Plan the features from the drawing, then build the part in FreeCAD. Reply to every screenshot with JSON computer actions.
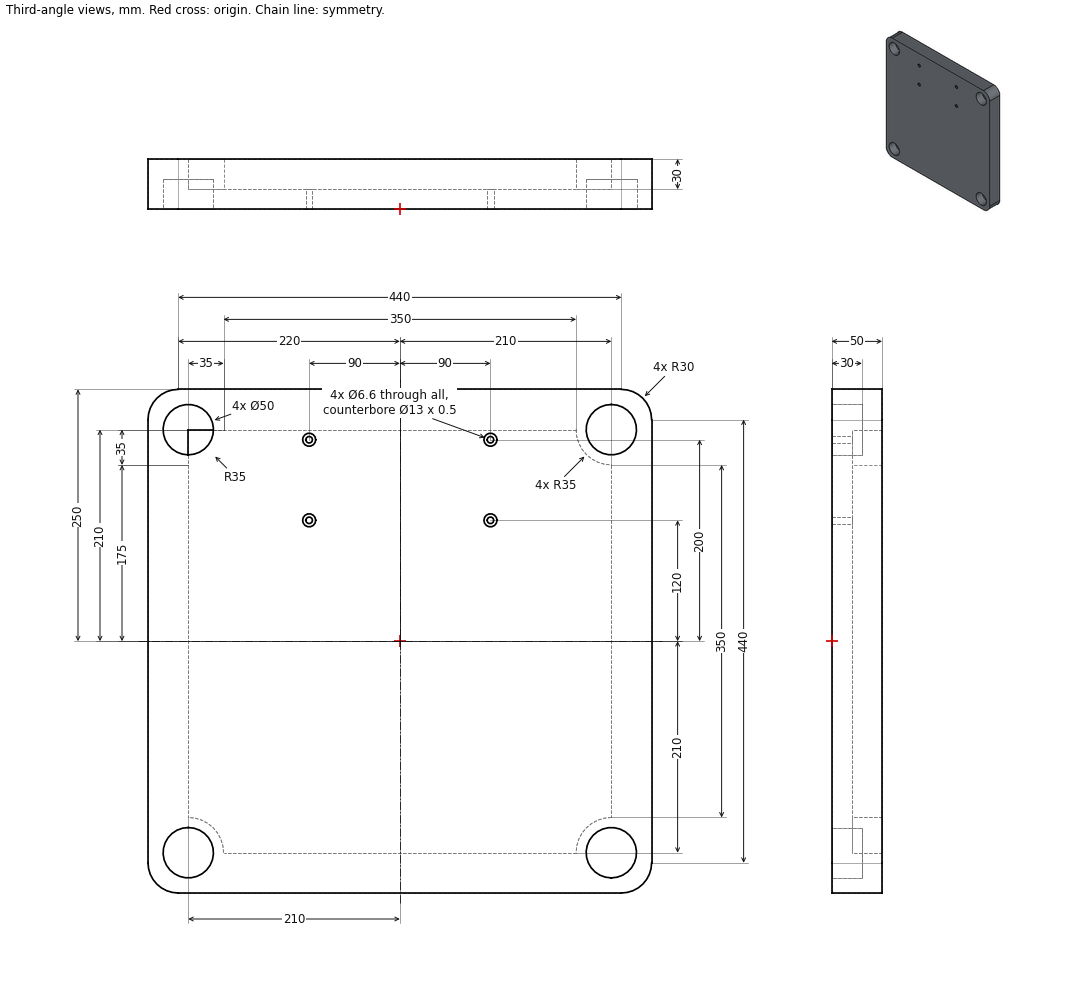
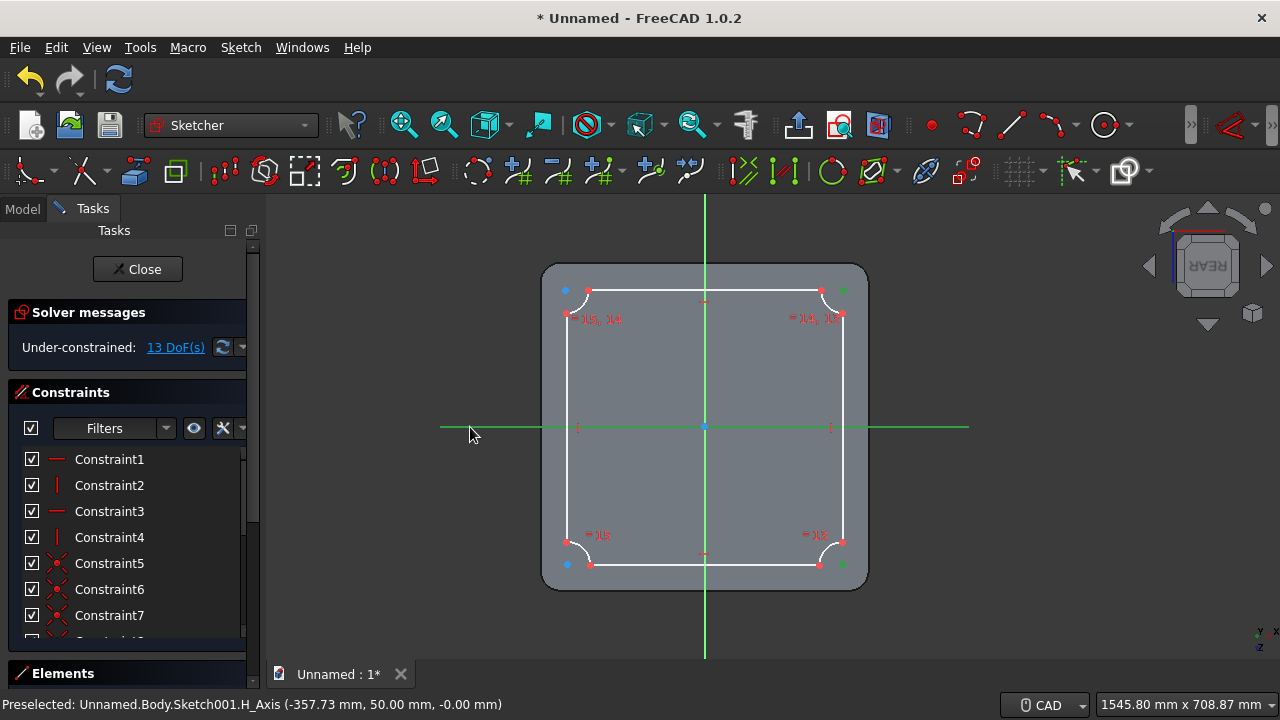
{"action": "key", "text": "s"}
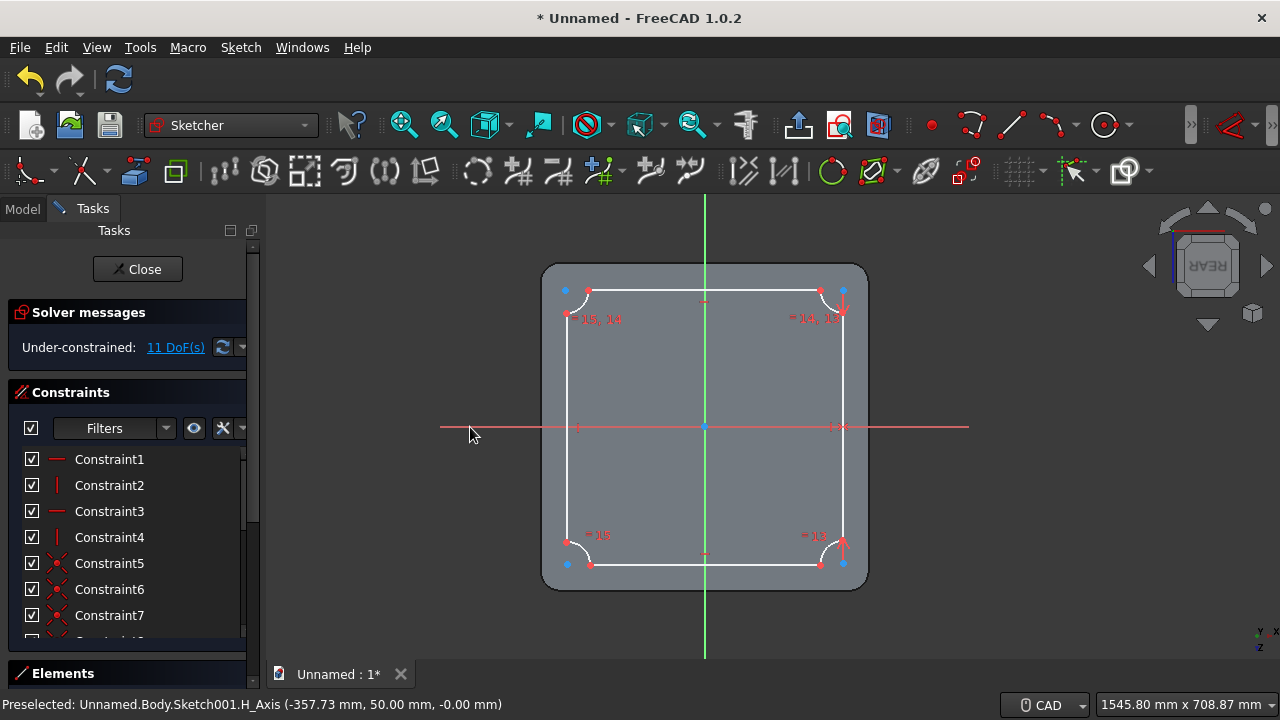
{"action": "left_click", "coordinate": [843, 290]}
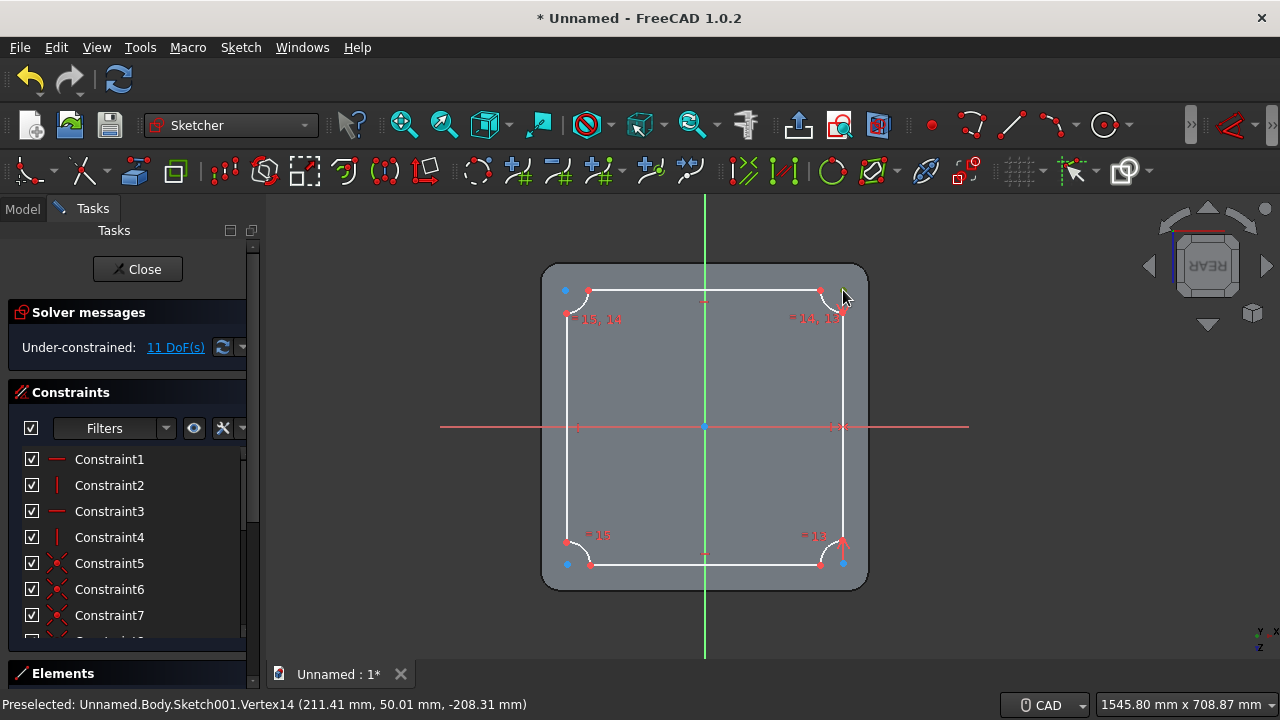
{"action": "left_click", "coordinate": [566, 291]}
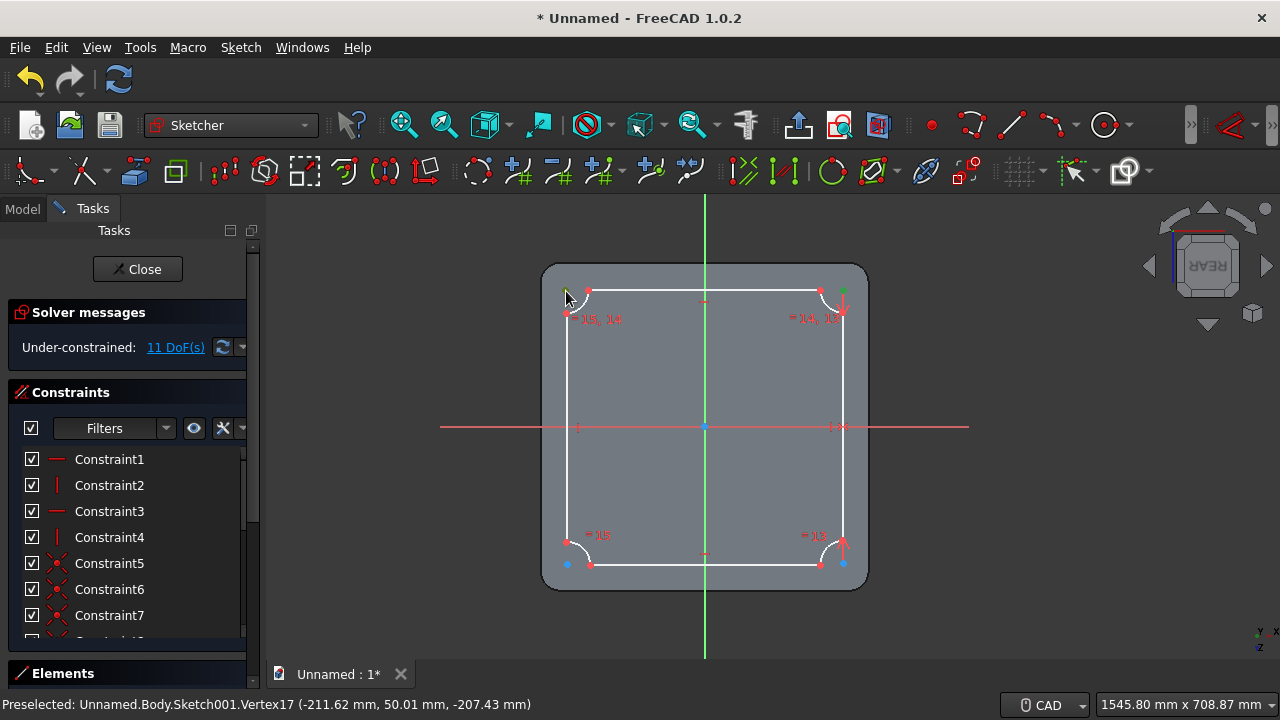
{"action": "left_click", "coordinate": [705, 602]}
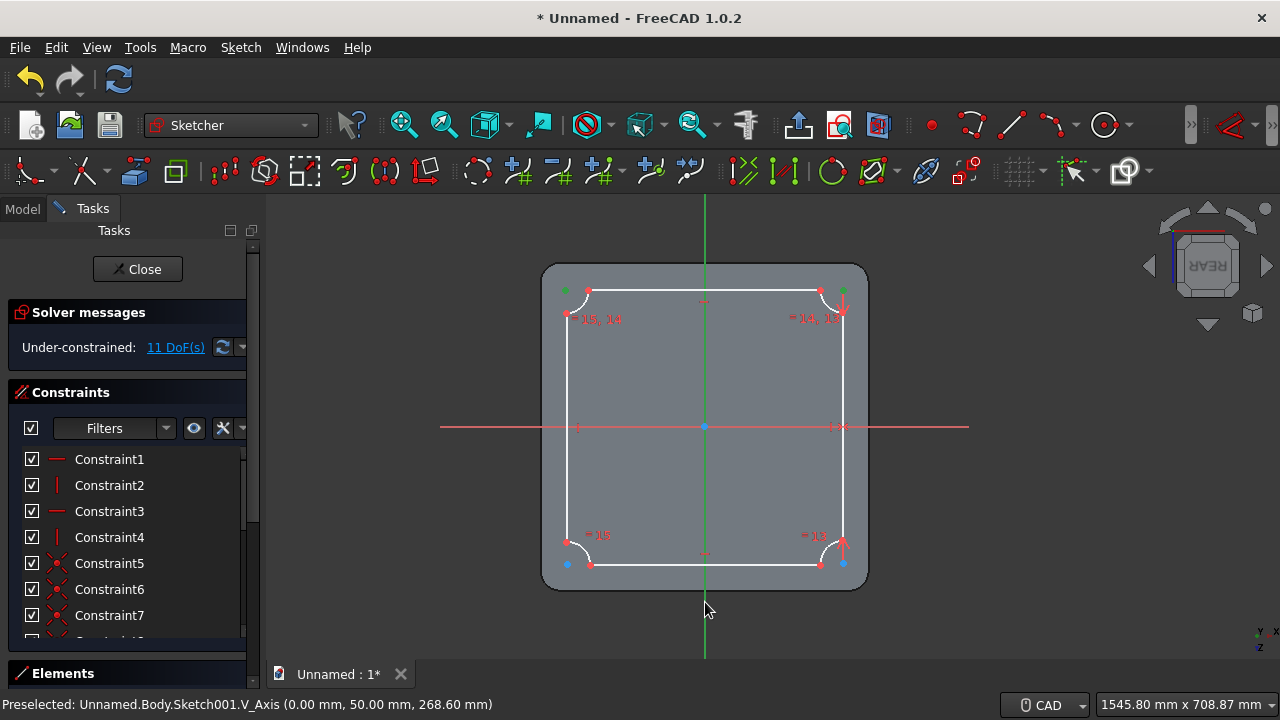
{"action": "key", "text": "s"}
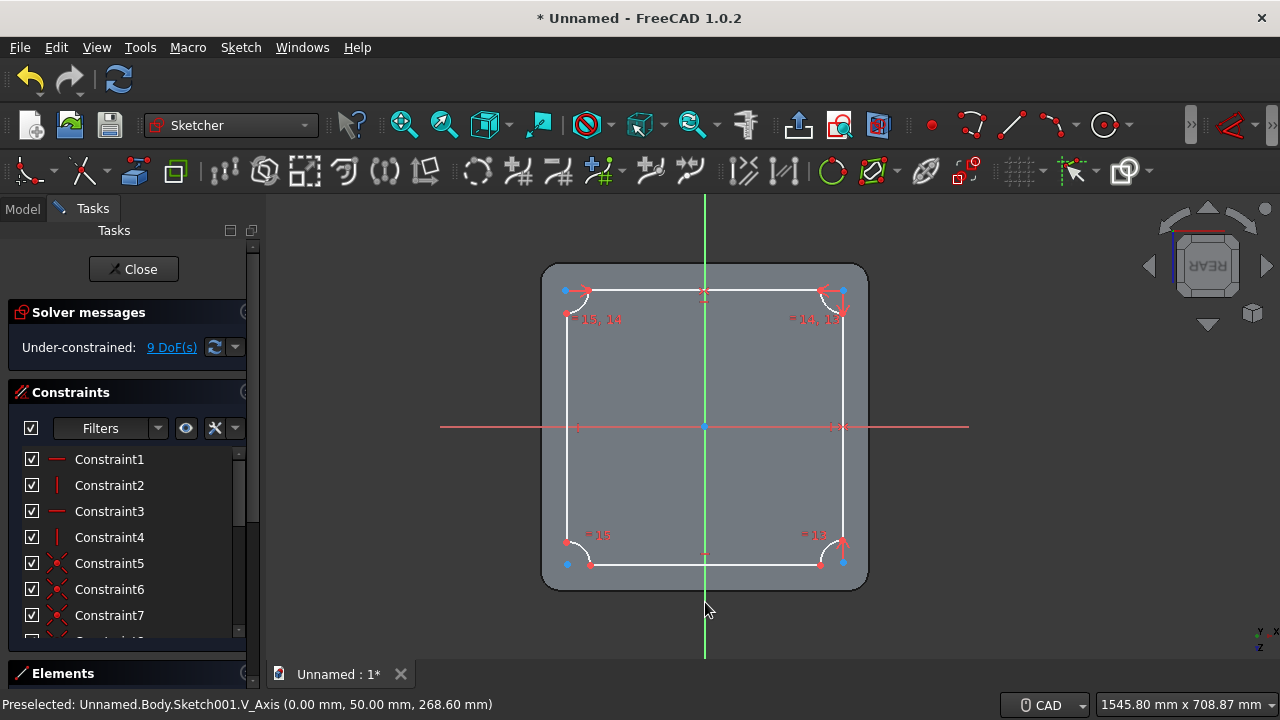
{"action": "left_click", "coordinate": [843, 563]}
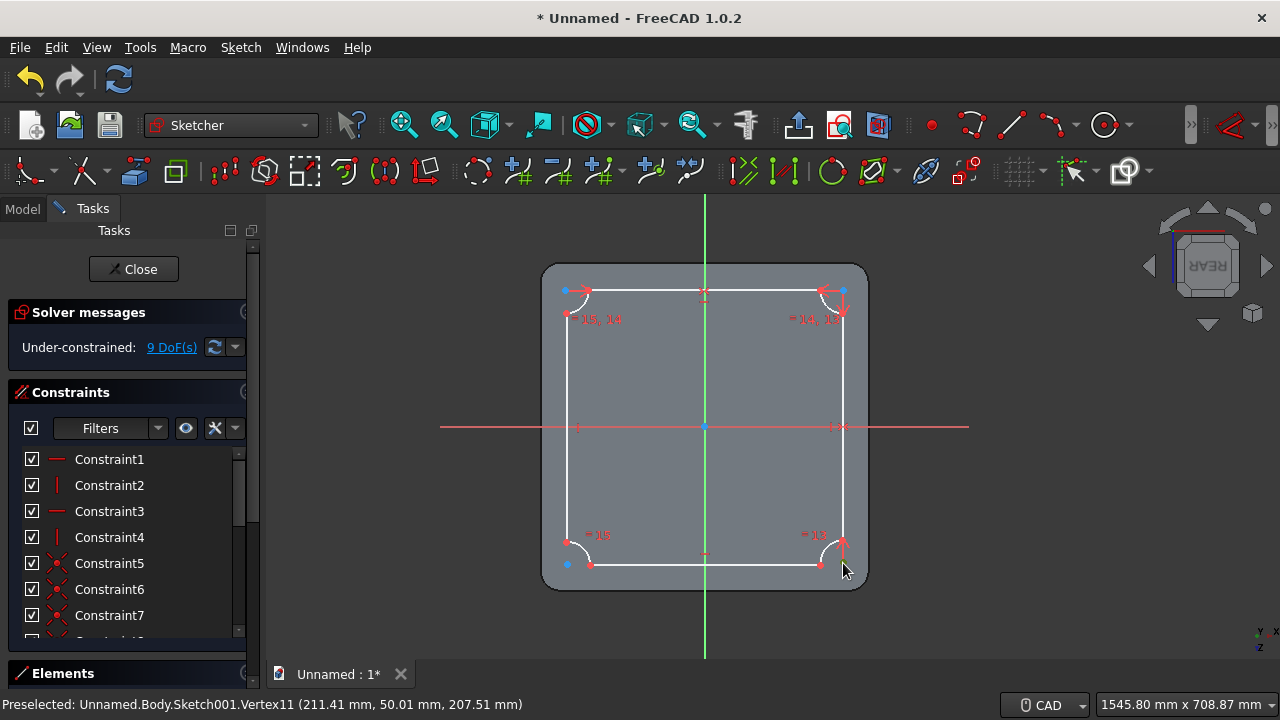
{"action": "left_click", "coordinate": [567, 565]}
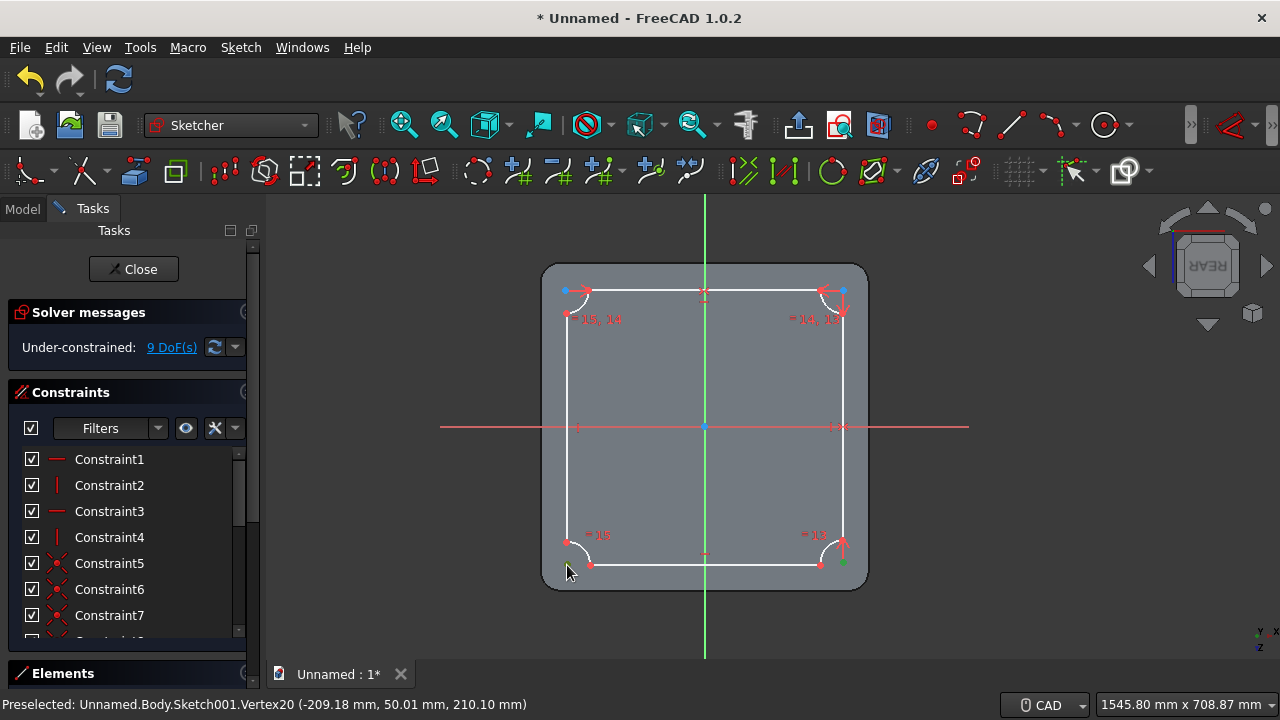
{"action": "left_click", "coordinate": [705, 602]}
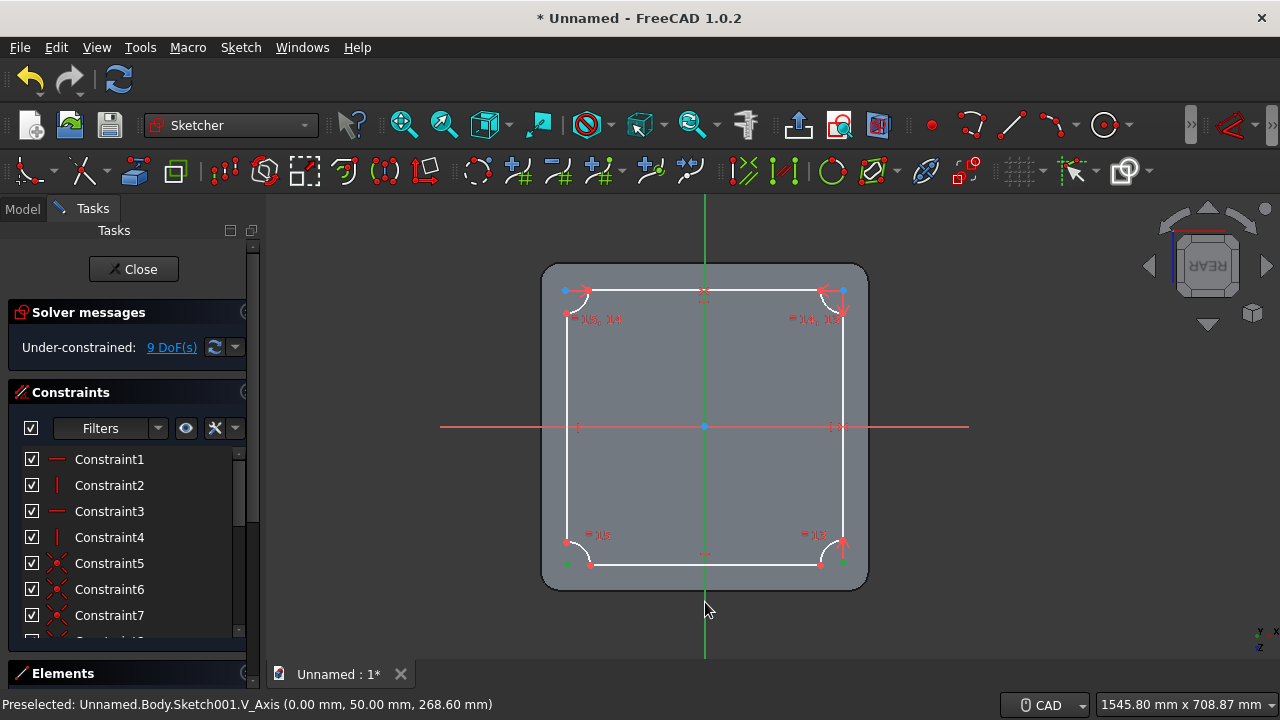
{"action": "key", "text": "s"}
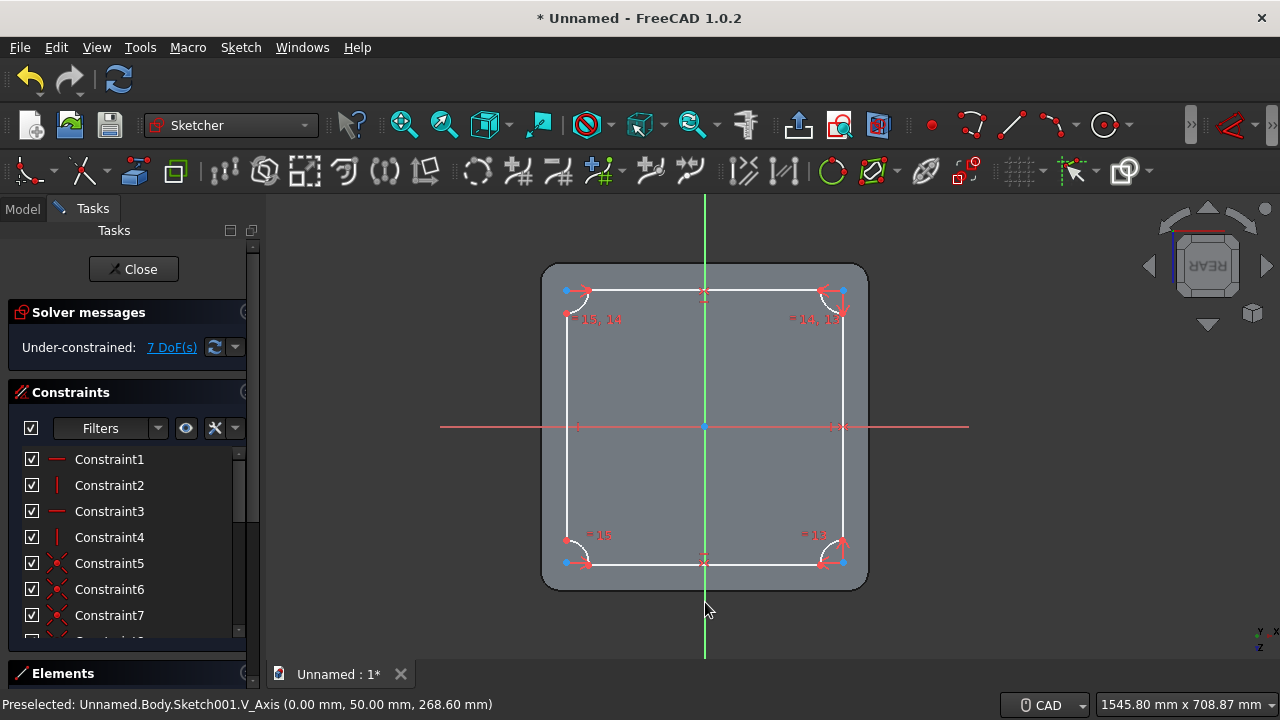
{"action": "key", "text": "d"}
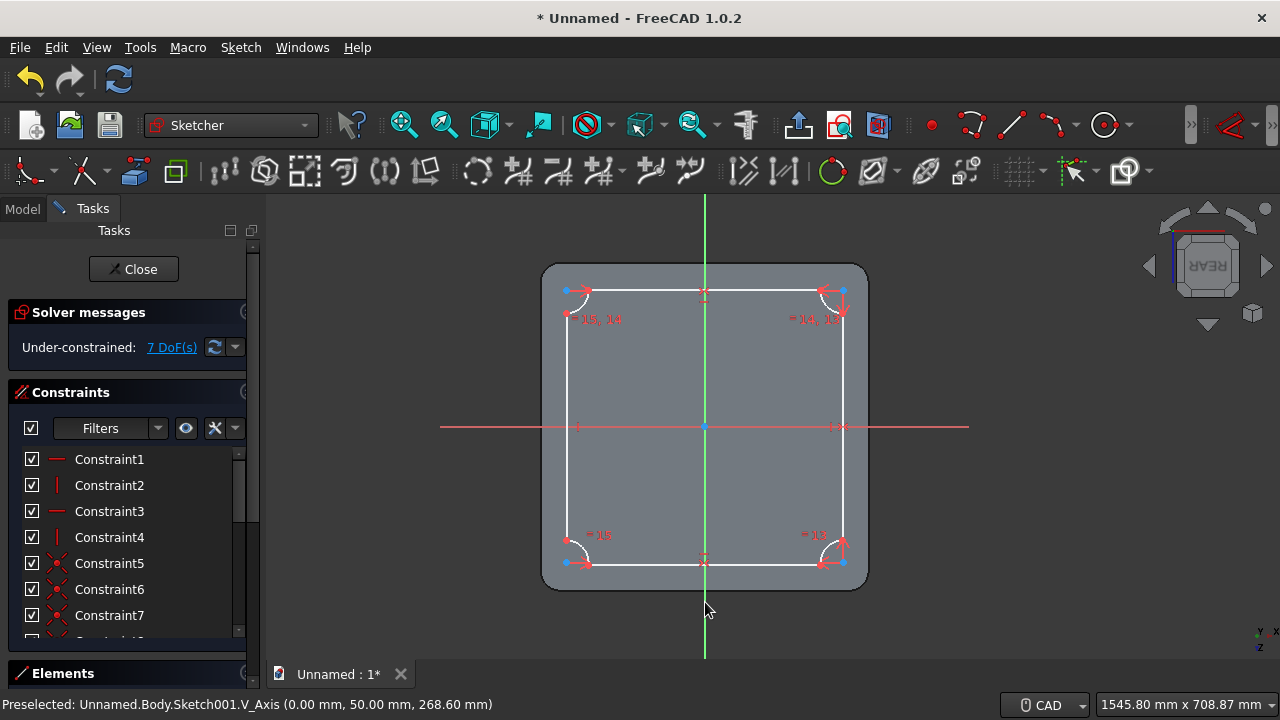
{"action": "scroll", "coordinate": [832, 543], "scroll_direction": "up", "scroll_amount": 3}